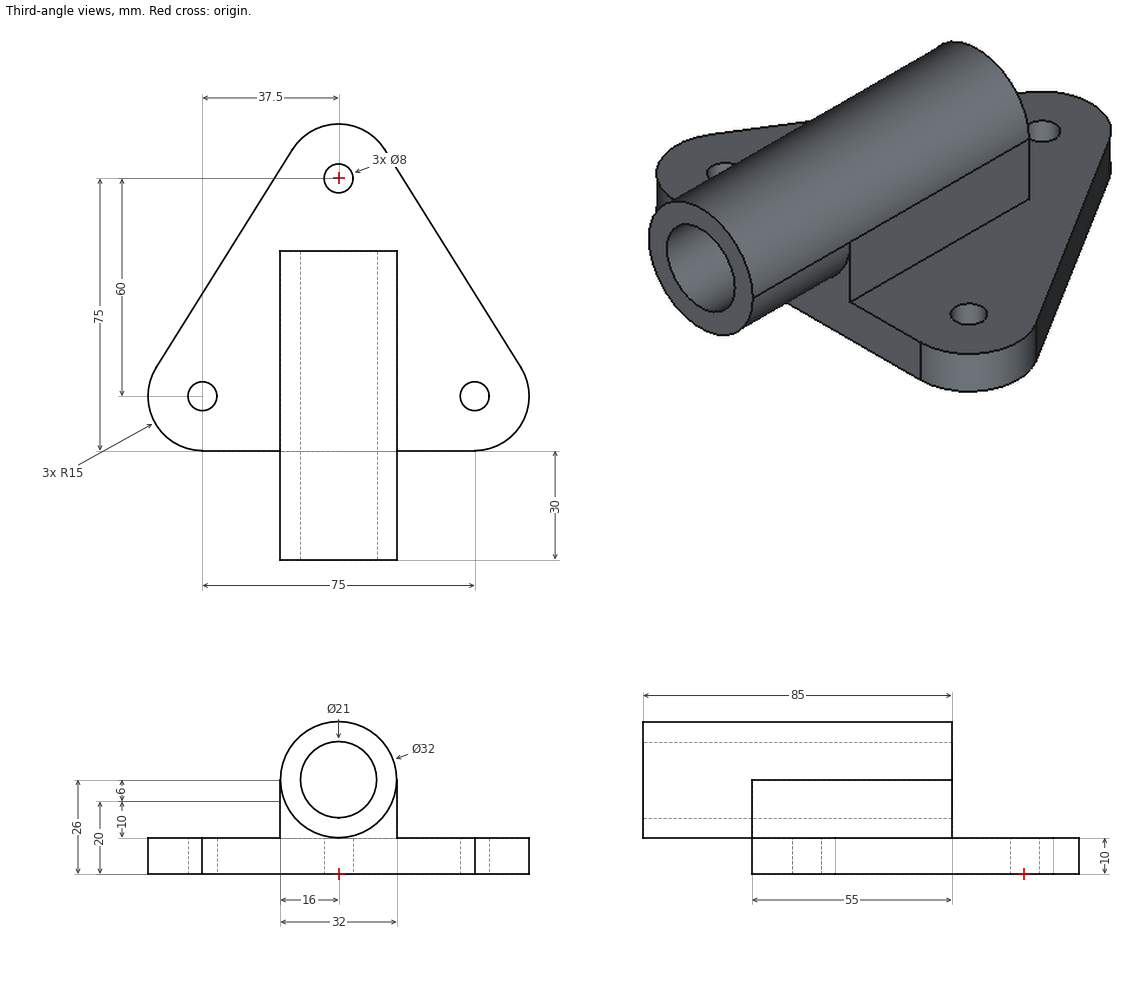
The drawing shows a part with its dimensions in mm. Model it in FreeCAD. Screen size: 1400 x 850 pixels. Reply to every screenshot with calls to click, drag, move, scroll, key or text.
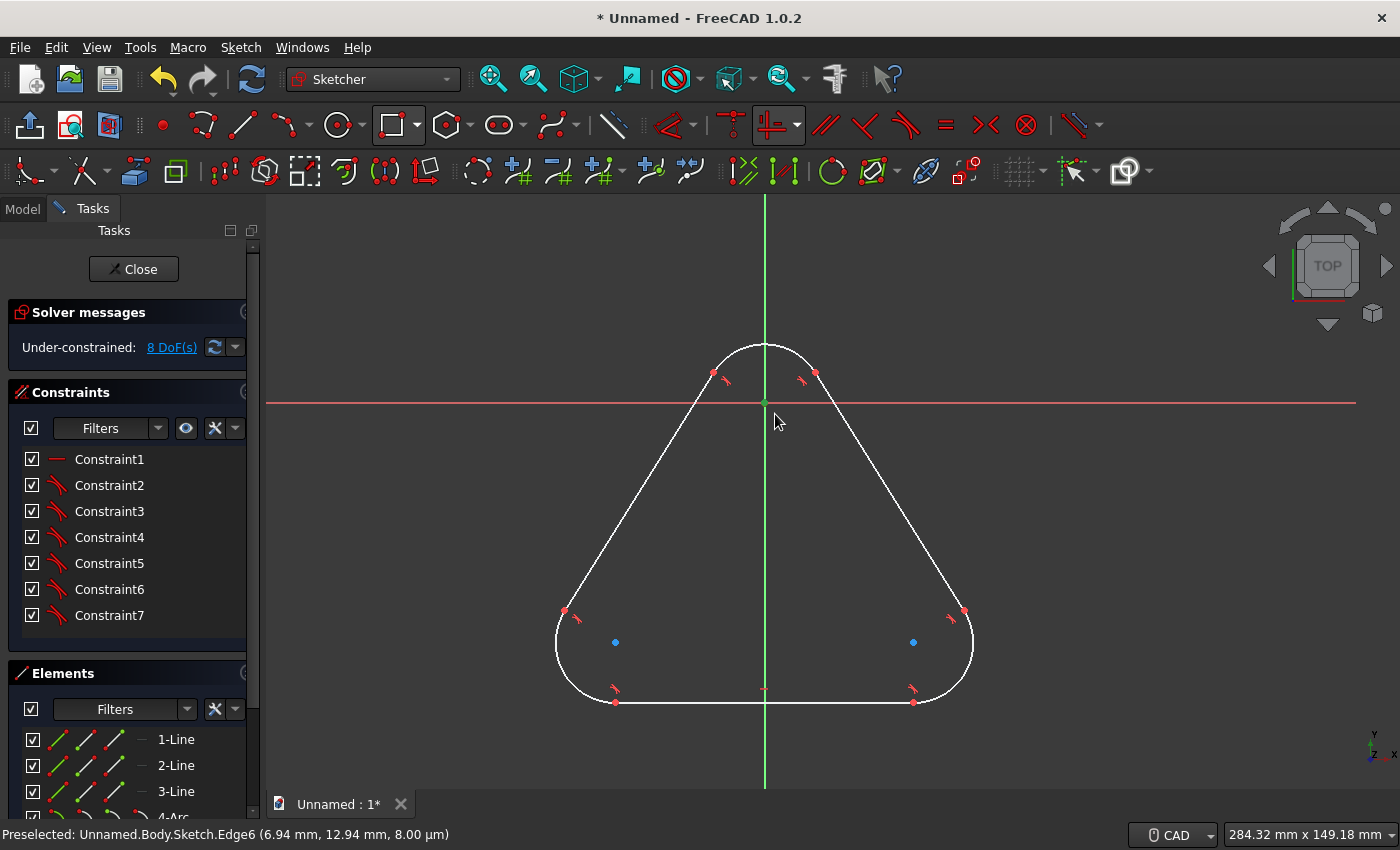
click(732, 126)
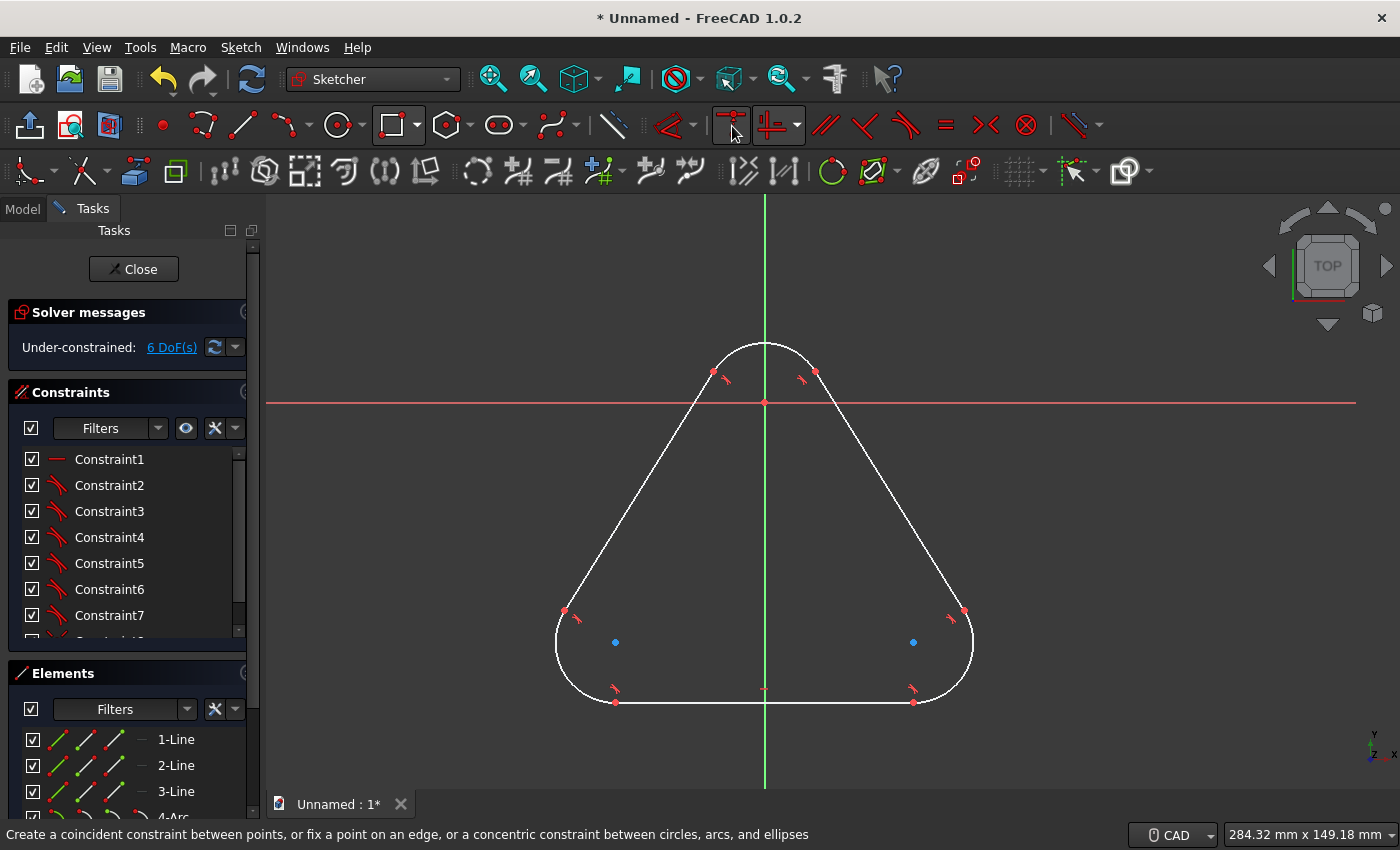
click(556, 648)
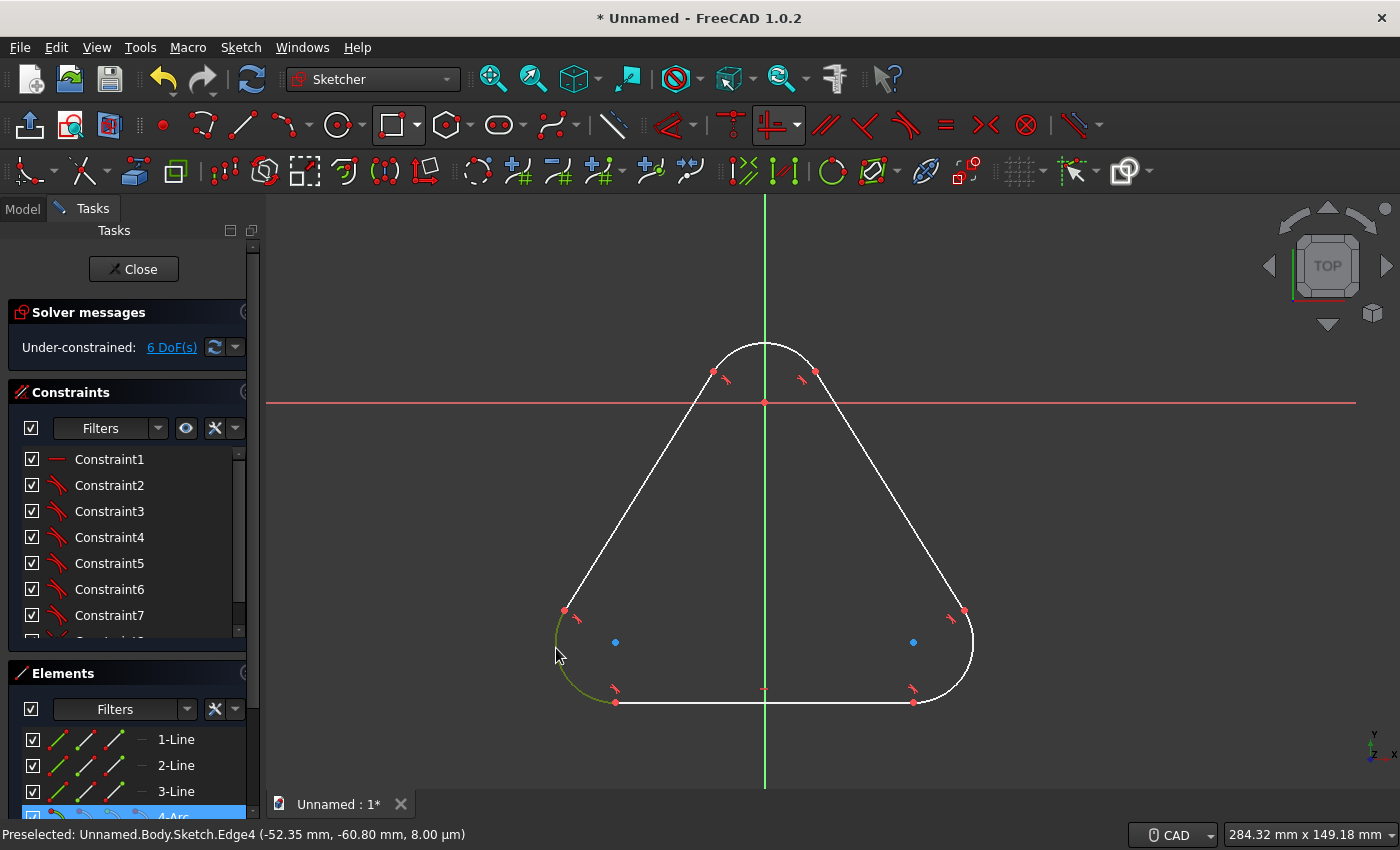
click(949, 691)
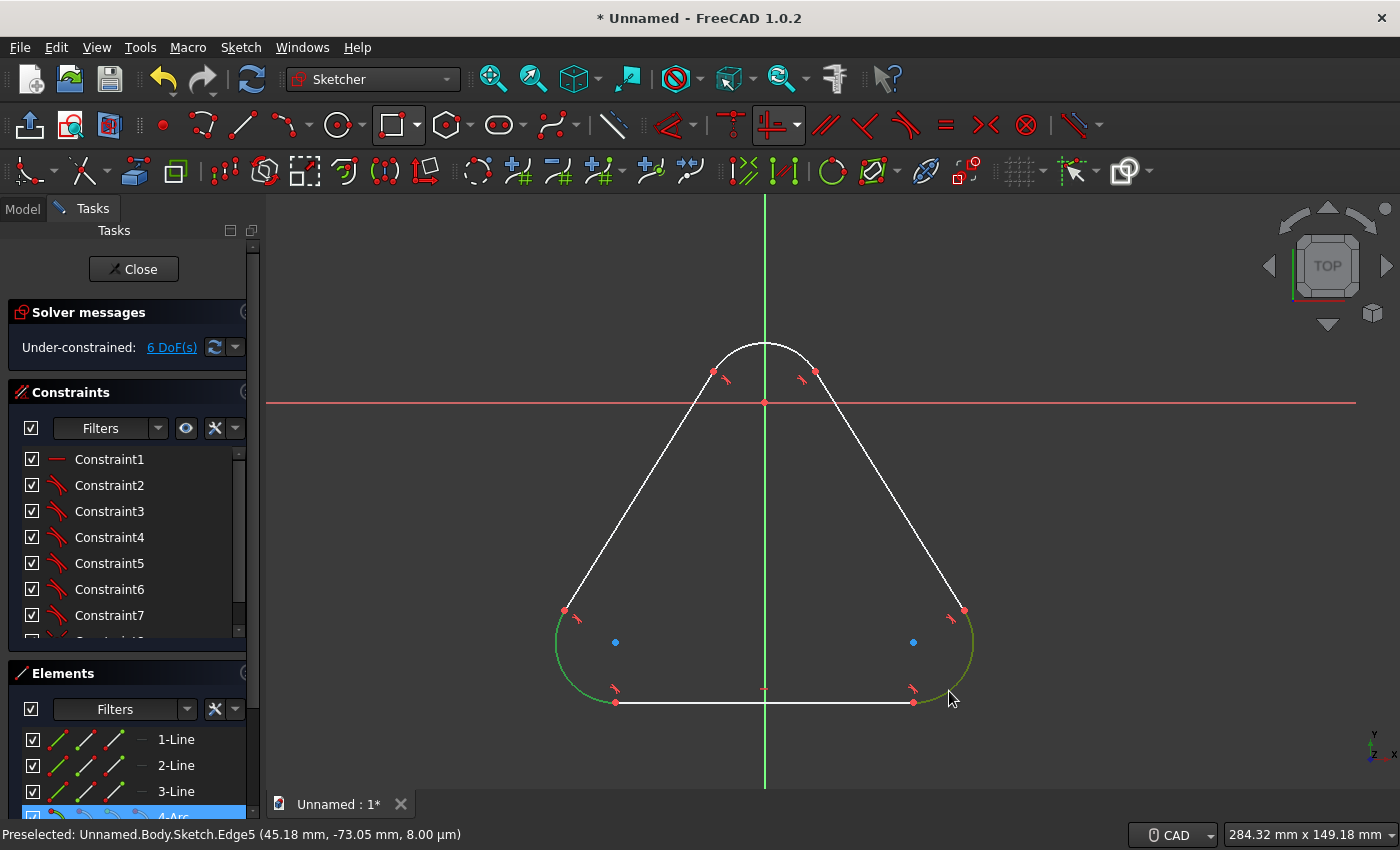
click(788, 348)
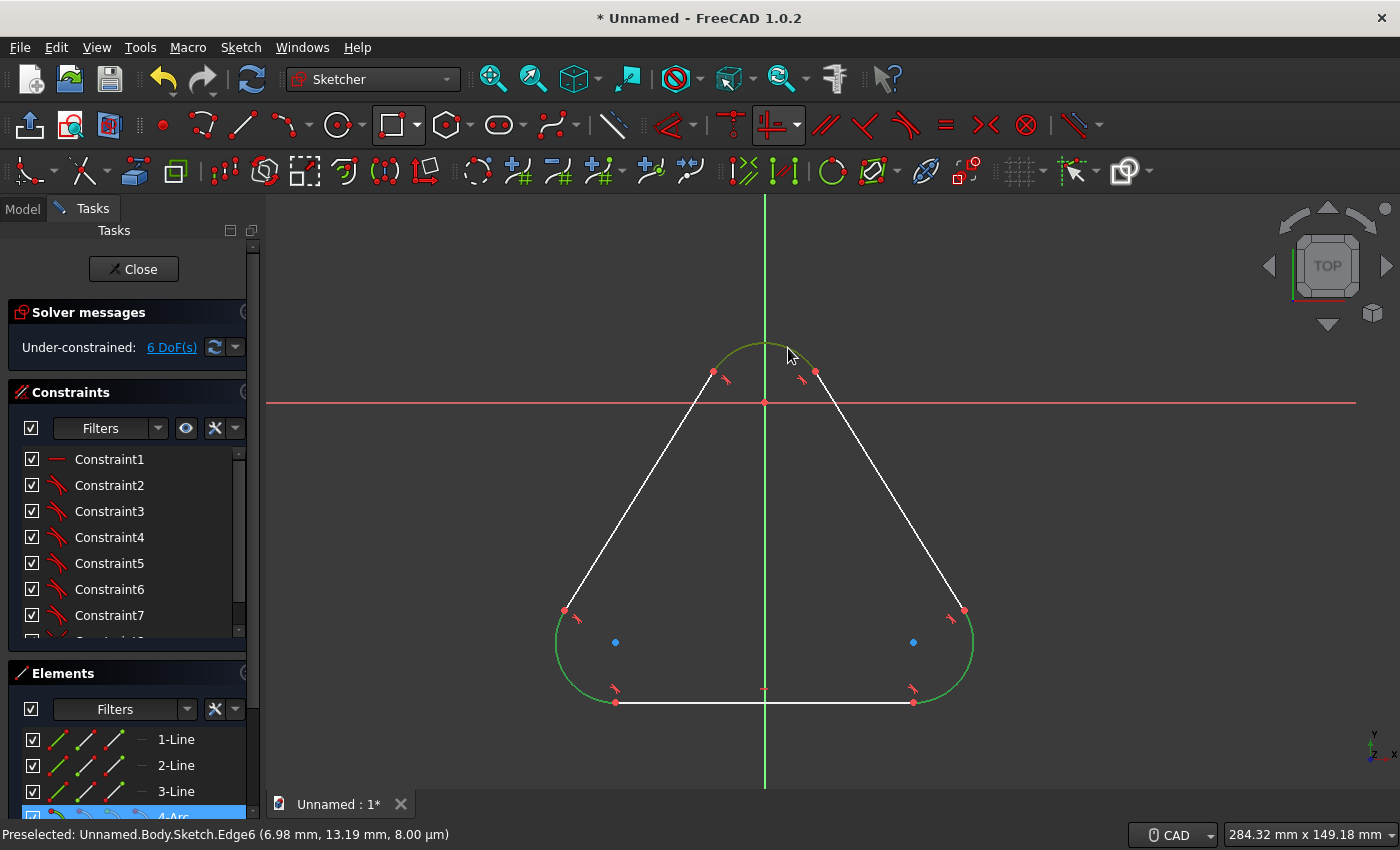
click(946, 126)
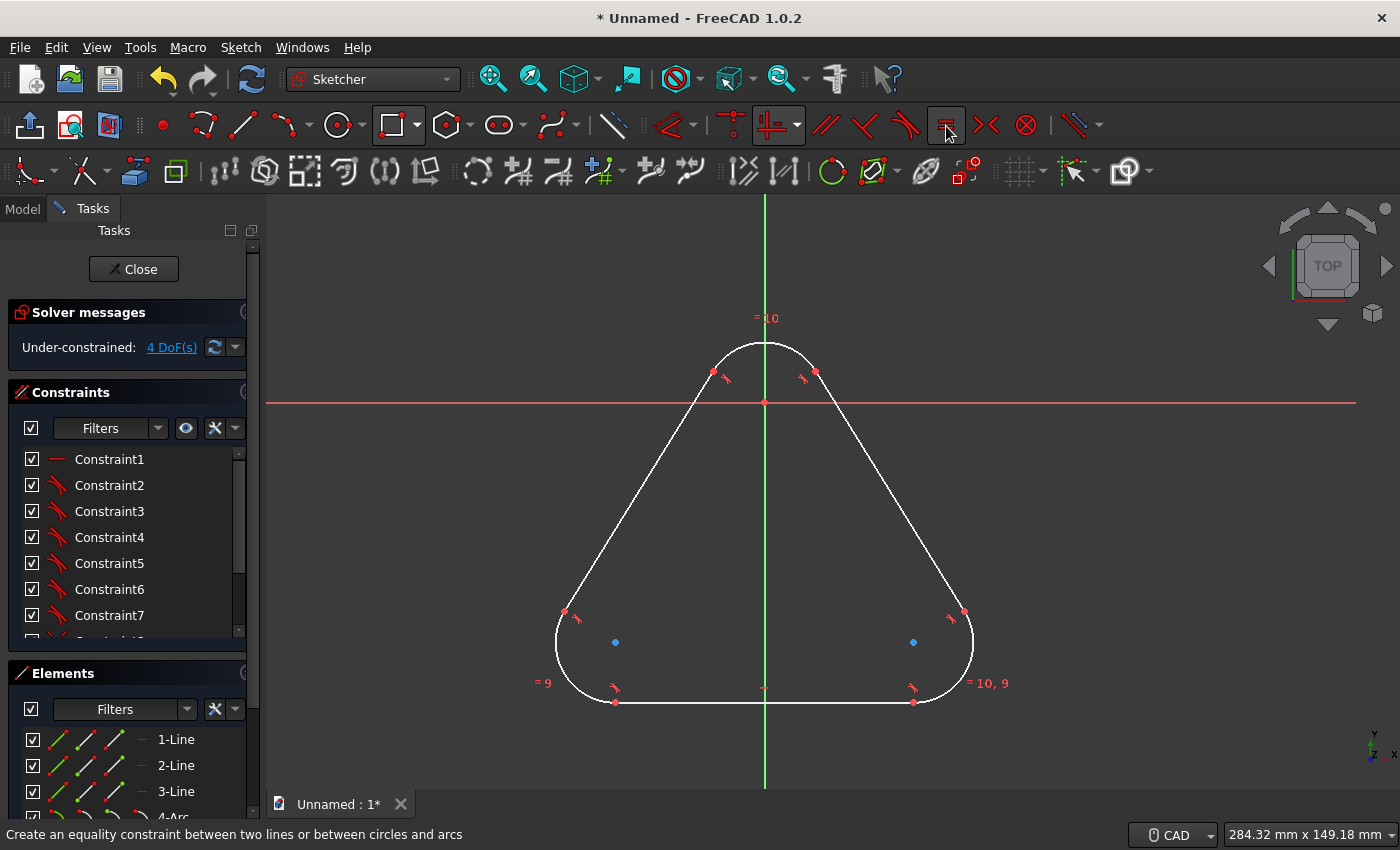
click(556, 648)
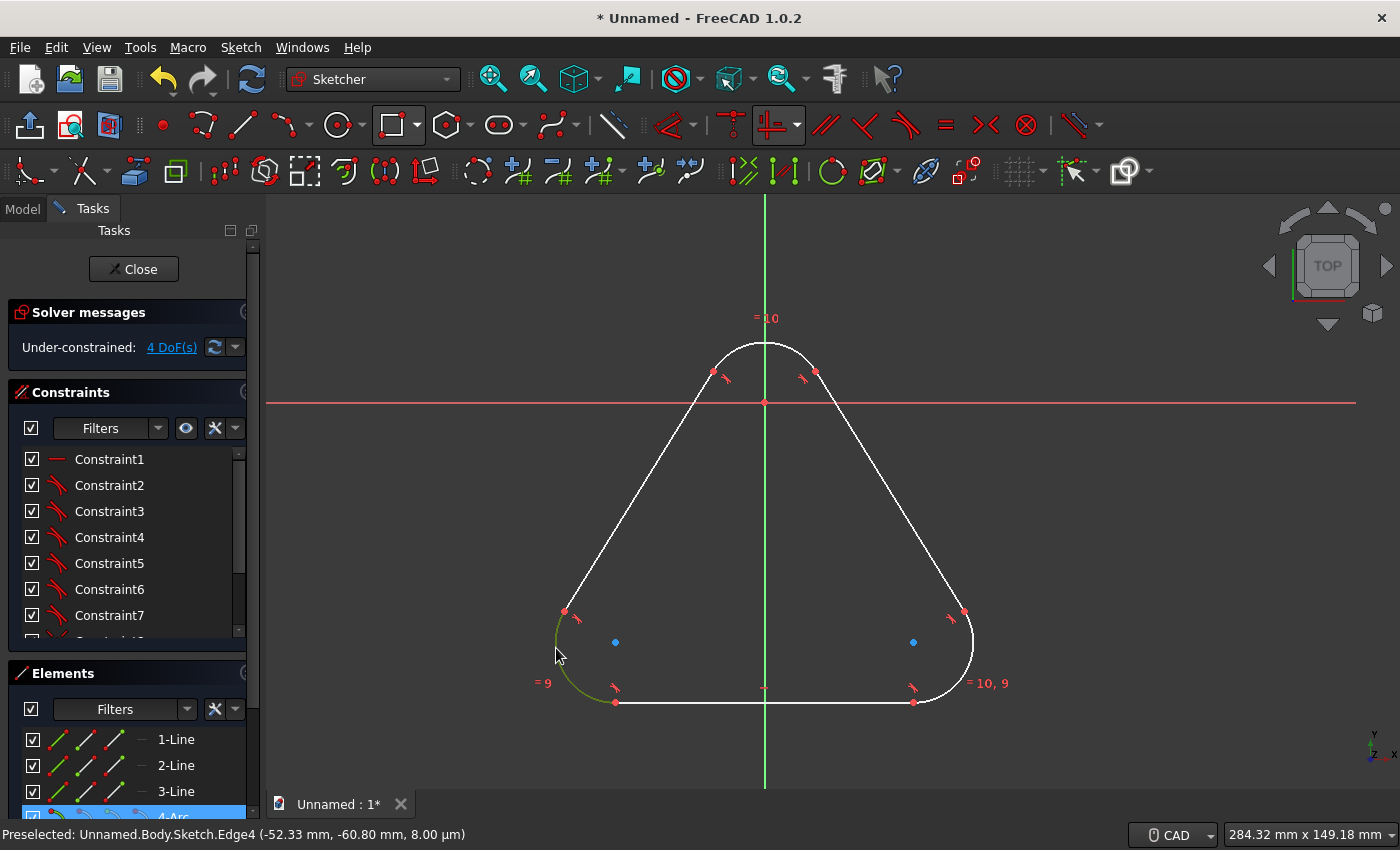
click(696, 126)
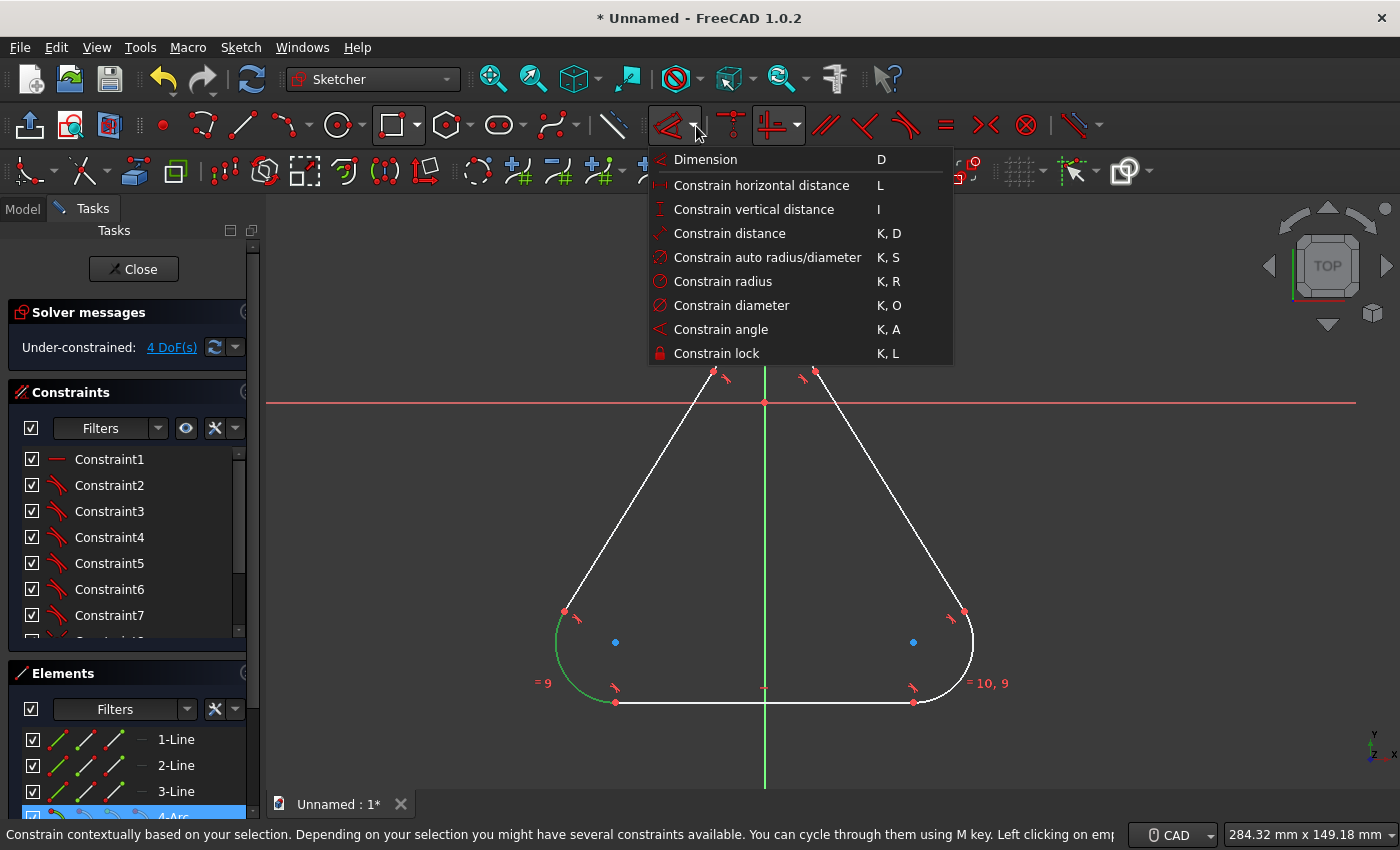
click(801, 281)